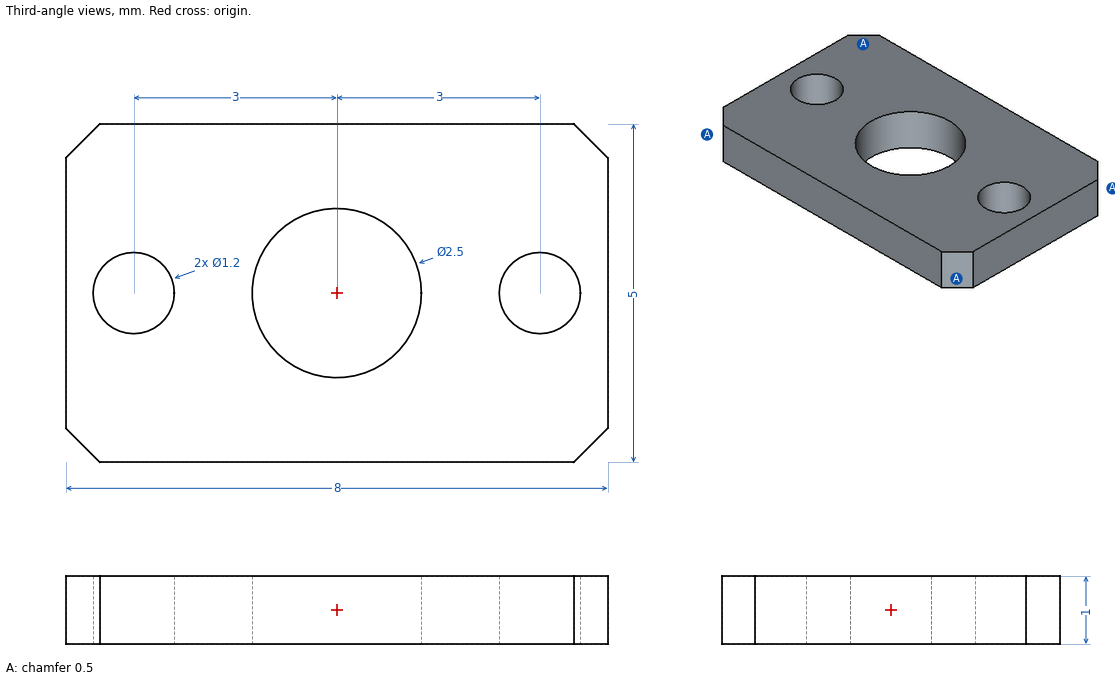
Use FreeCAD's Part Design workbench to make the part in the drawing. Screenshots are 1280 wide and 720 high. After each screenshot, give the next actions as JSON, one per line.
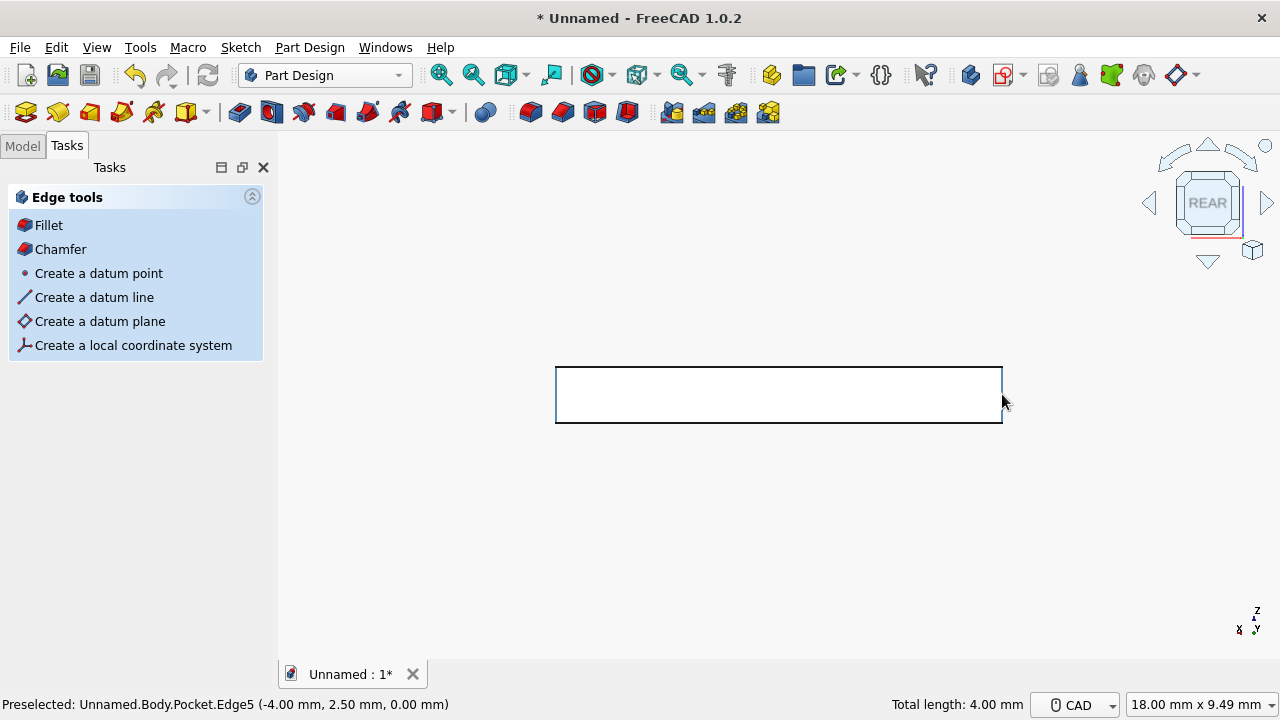
{"action": "left_click", "coordinate": [564, 112]}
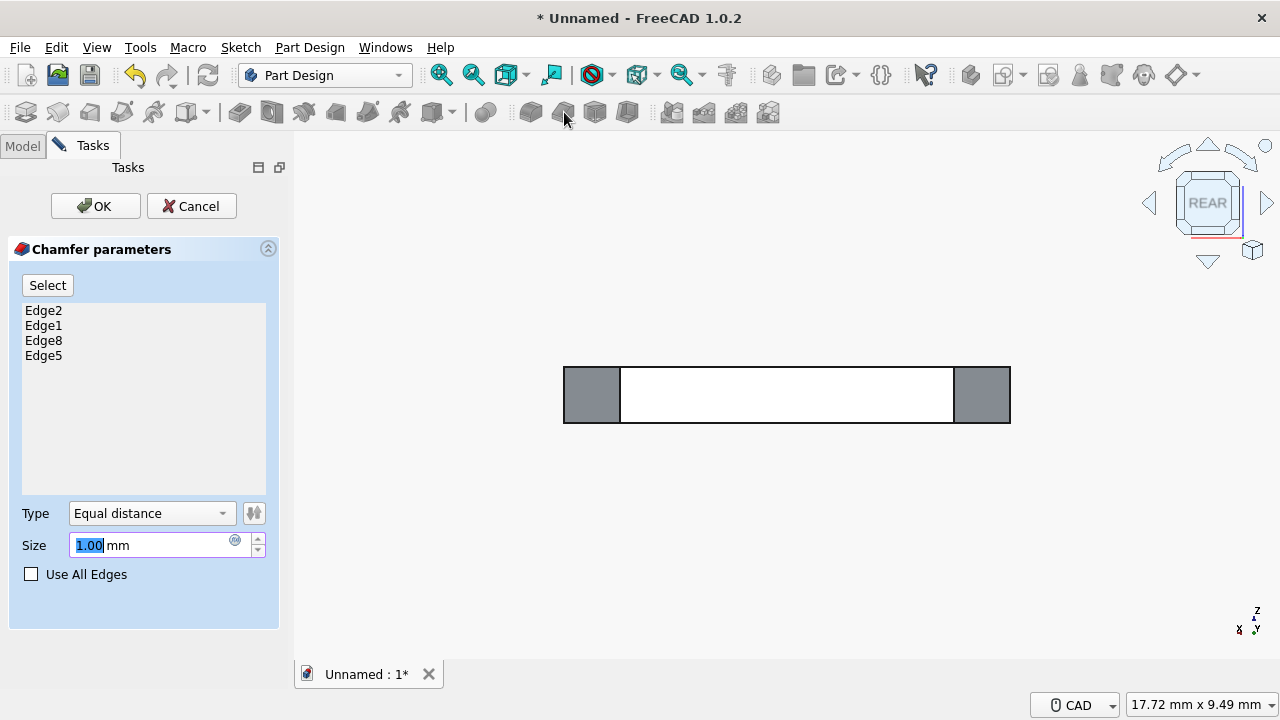
{"action": "type", "text": "0.5"}
{"action": "key", "text": "Tab"}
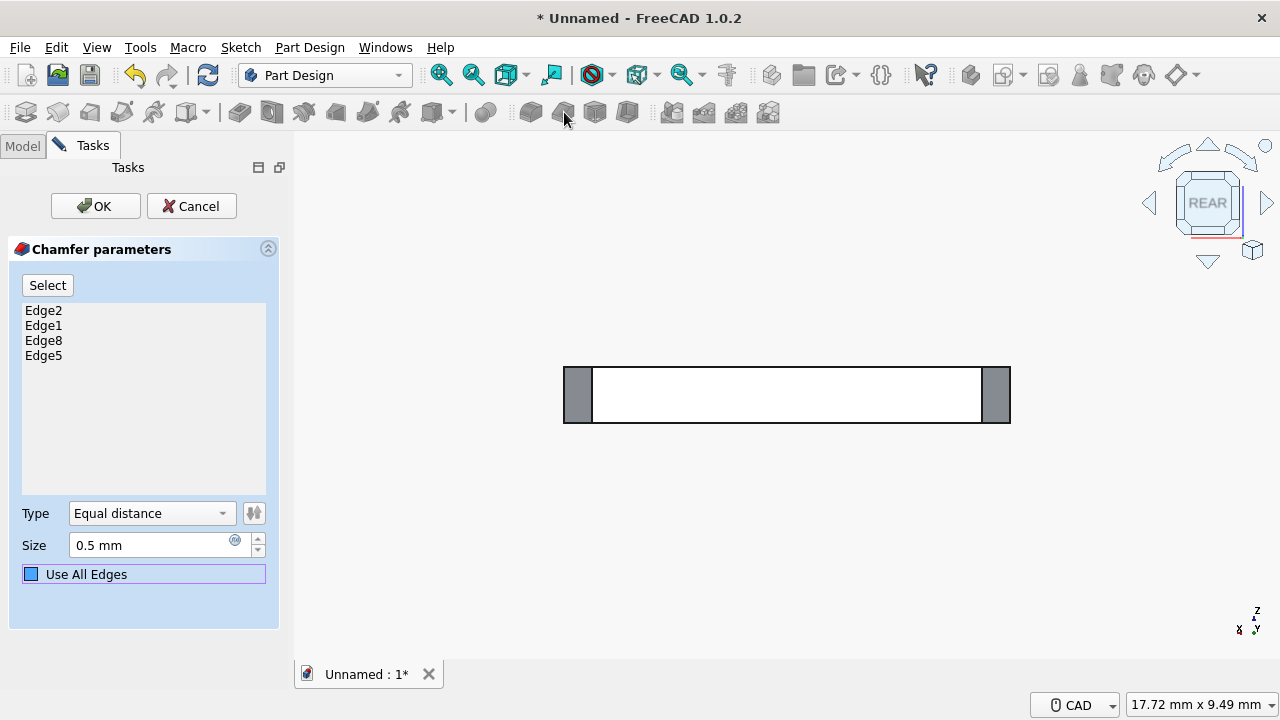
{"action": "left_click", "coordinate": [96, 206]}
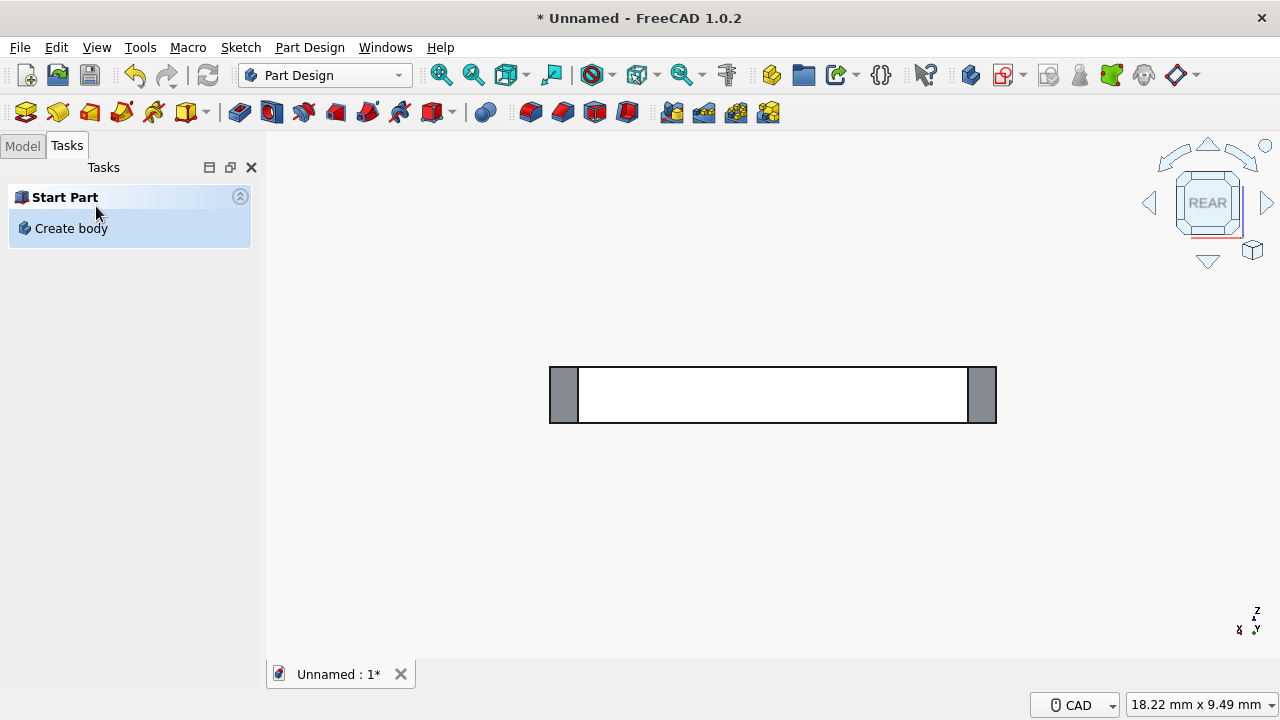
{"action": "key", "text": "0"}